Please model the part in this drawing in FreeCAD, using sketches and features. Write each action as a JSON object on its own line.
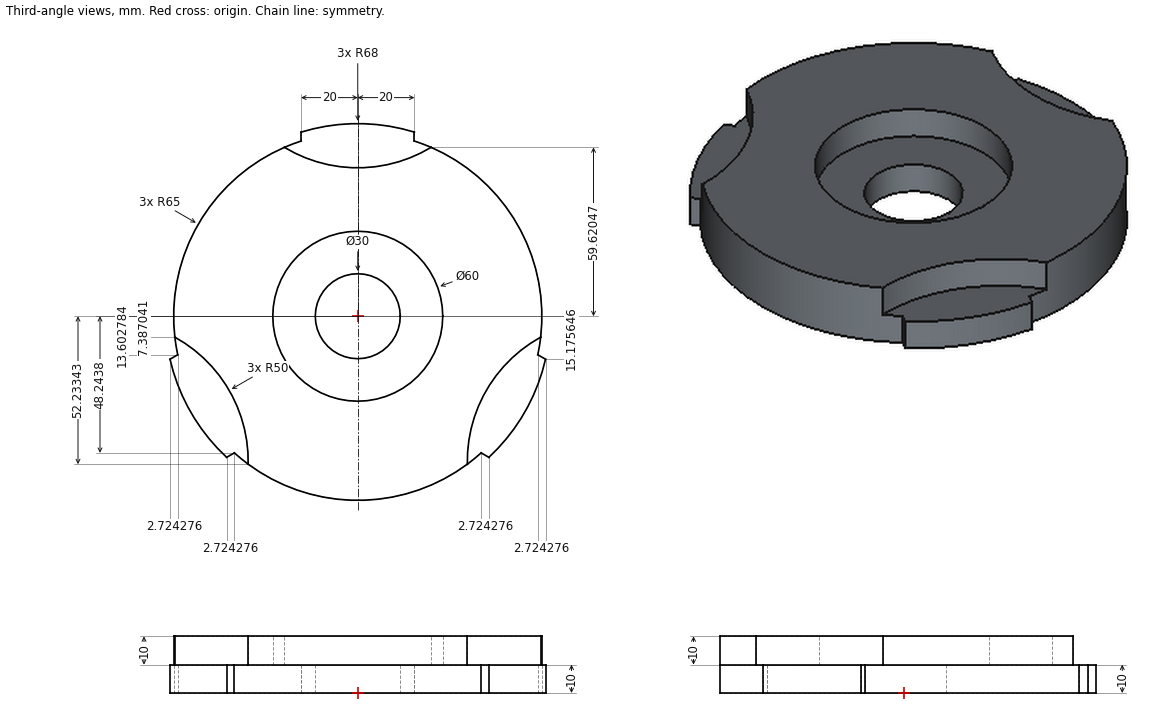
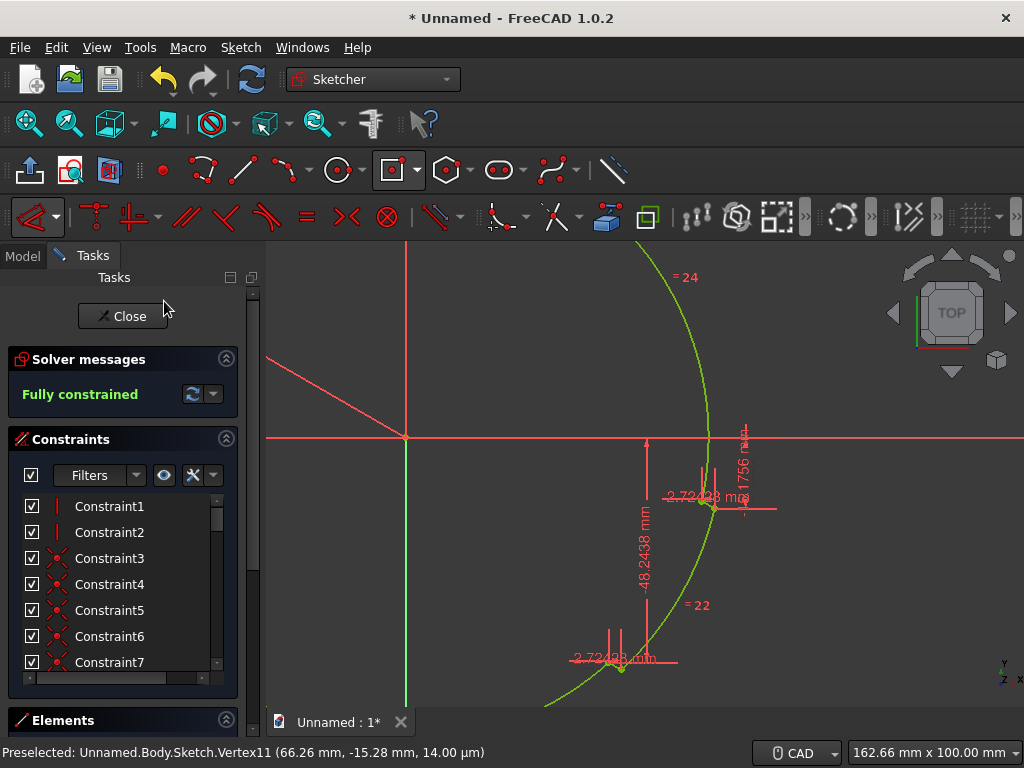
{"action": "left_click", "coordinate": [123, 316]}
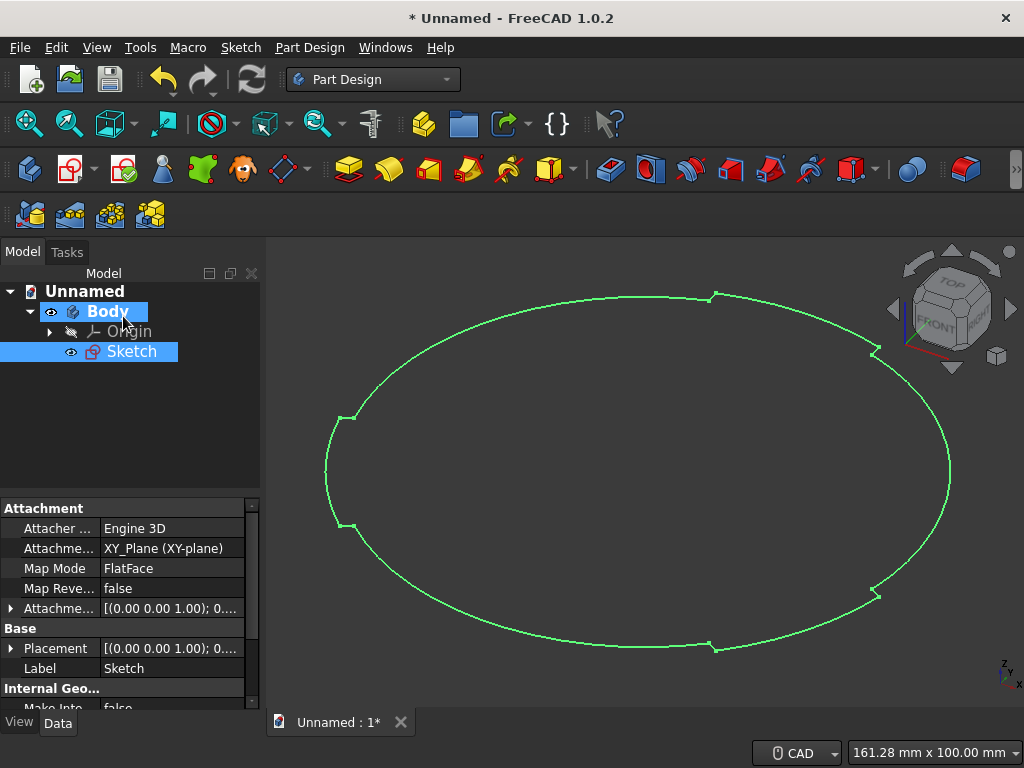
{"action": "left_click", "coordinate": [350, 170]}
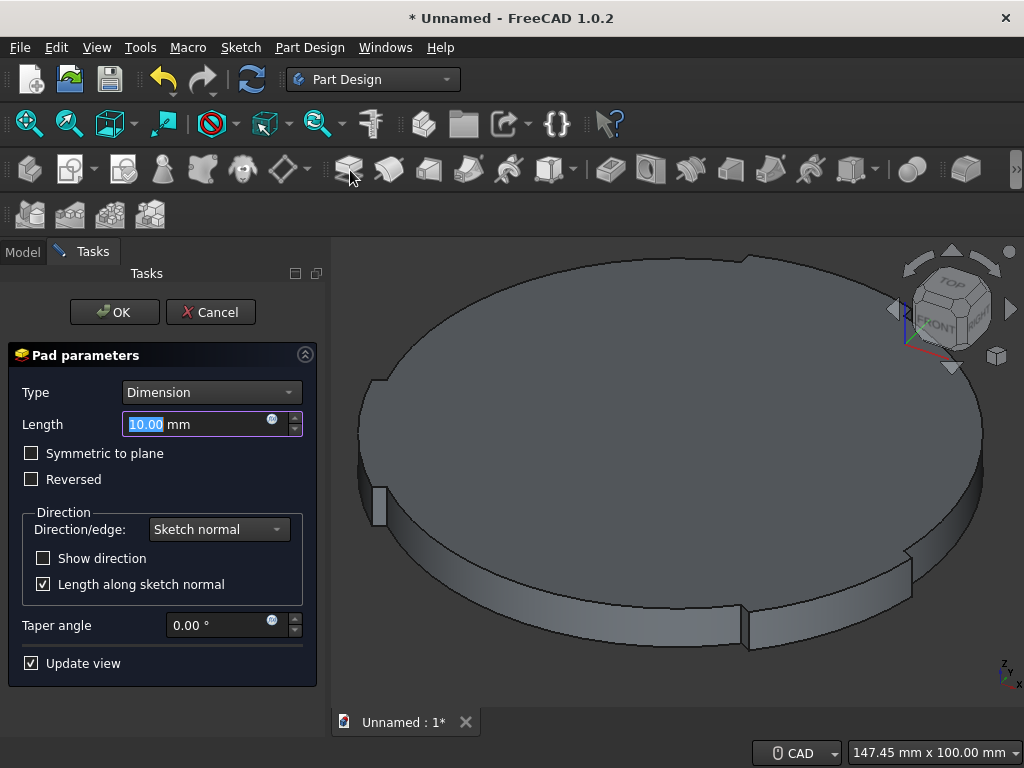
{"action": "type", "text": "10"}
{"action": "key", "text": "Tab"}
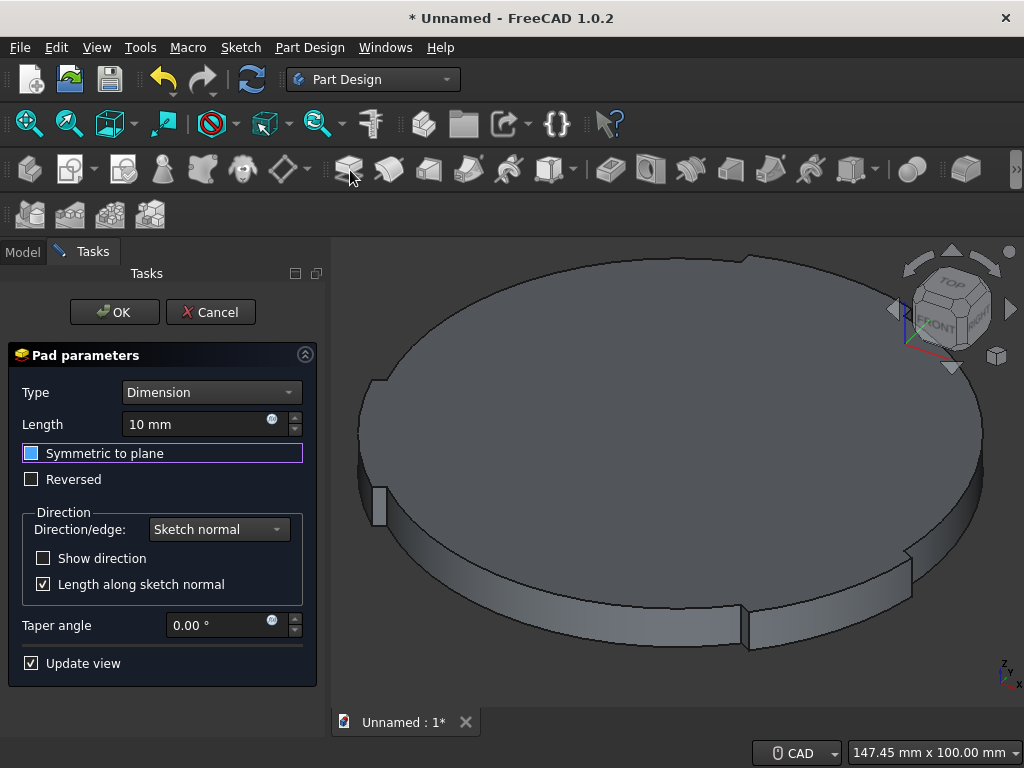
{"action": "left_click", "coordinate": [115, 312]}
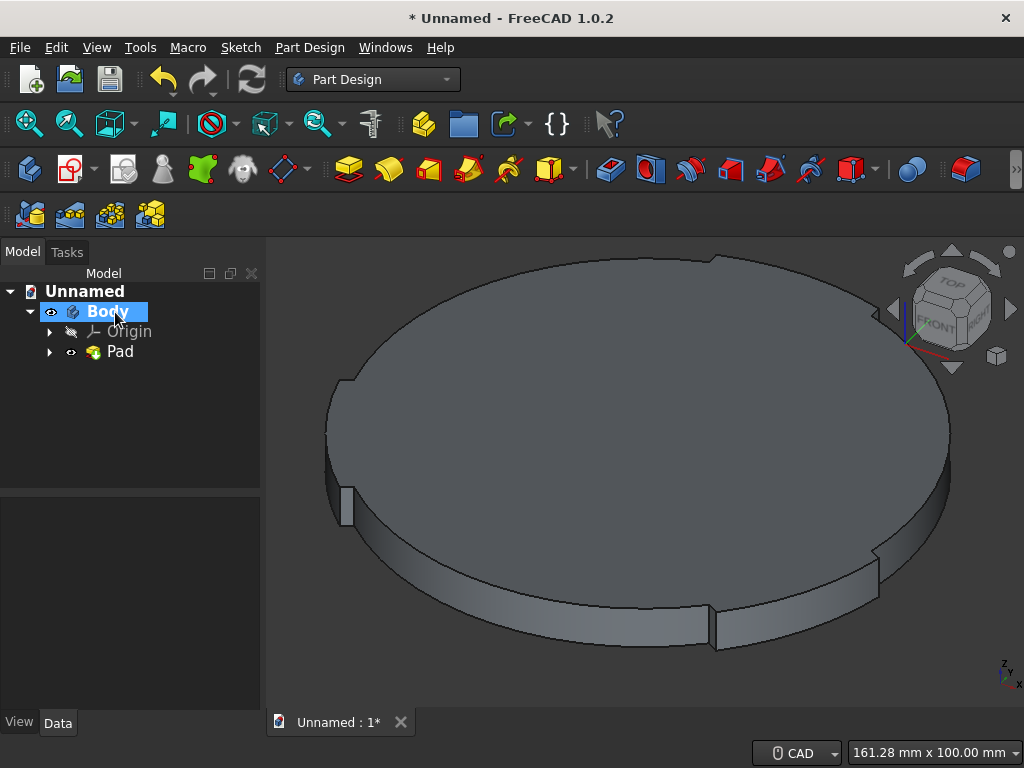
{"action": "left_click", "coordinate": [30, 124]}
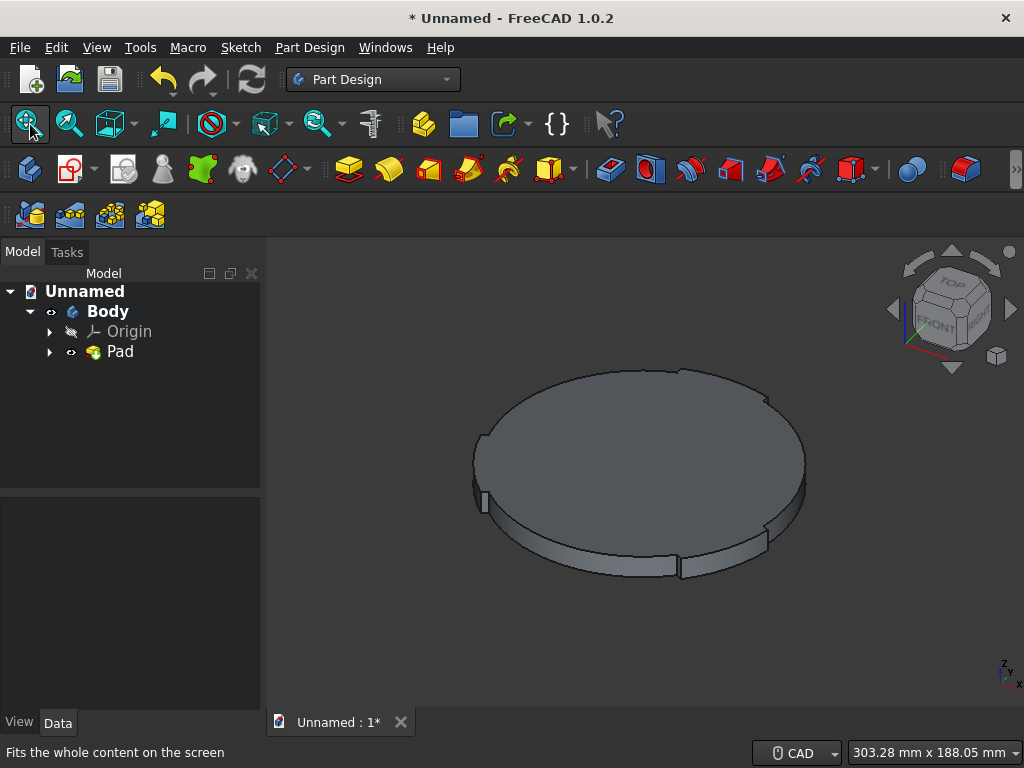
{"action": "left_click", "coordinate": [645, 461]}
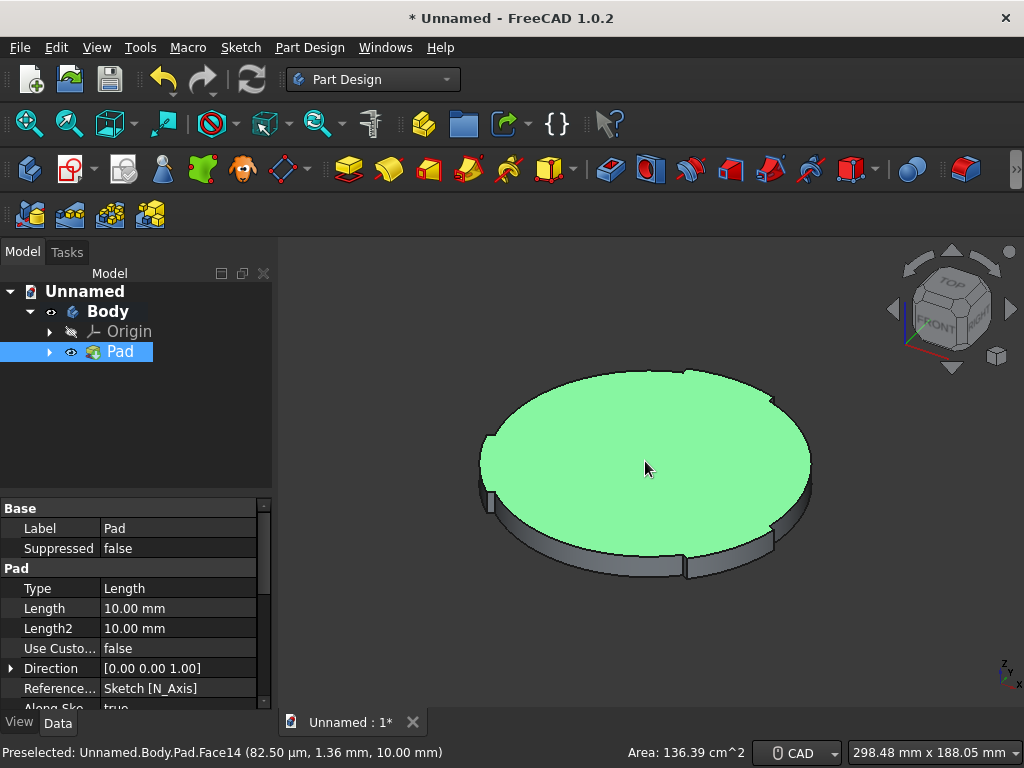
{"action": "left_click", "coordinate": [70, 170]}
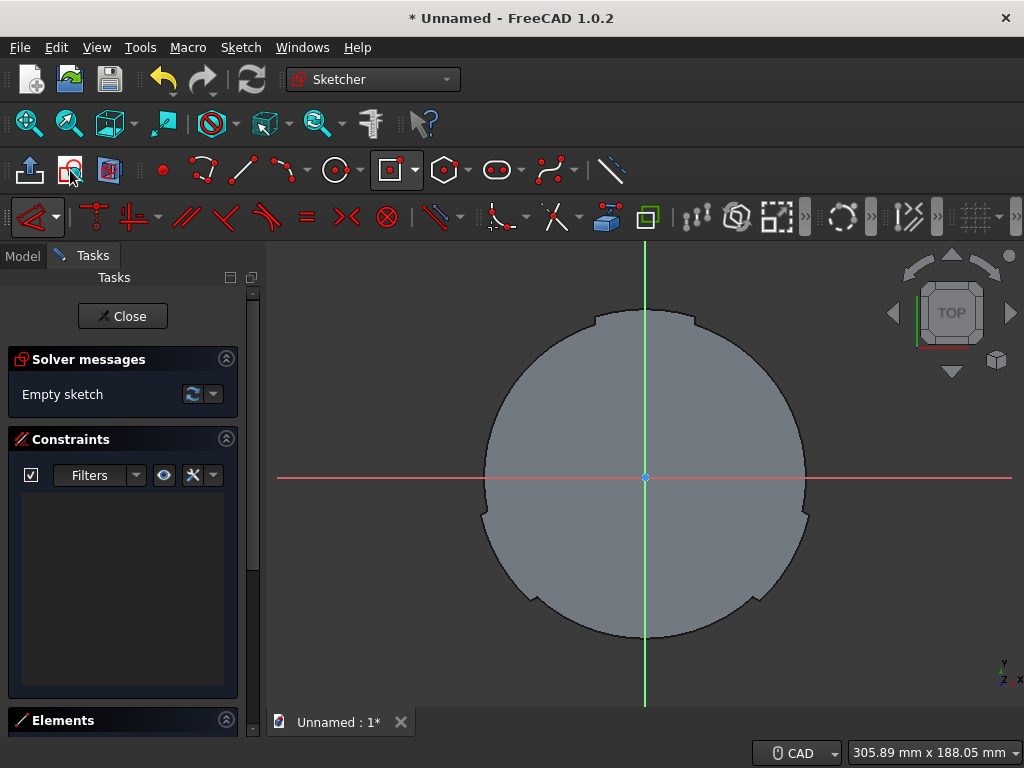
{"action": "left_click", "coordinate": [284, 170]}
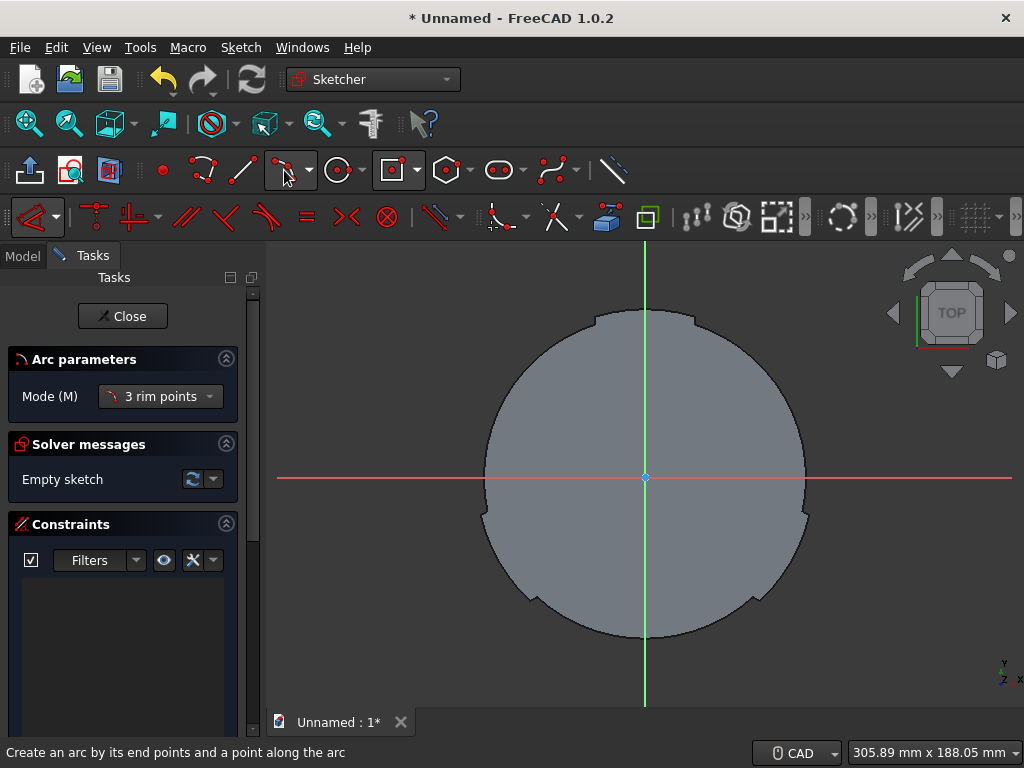
{"action": "left_click", "coordinate": [485, 496]}
{"action": "left_click", "coordinate": [549, 607]}
{"action": "left_click", "coordinate": [533, 543]}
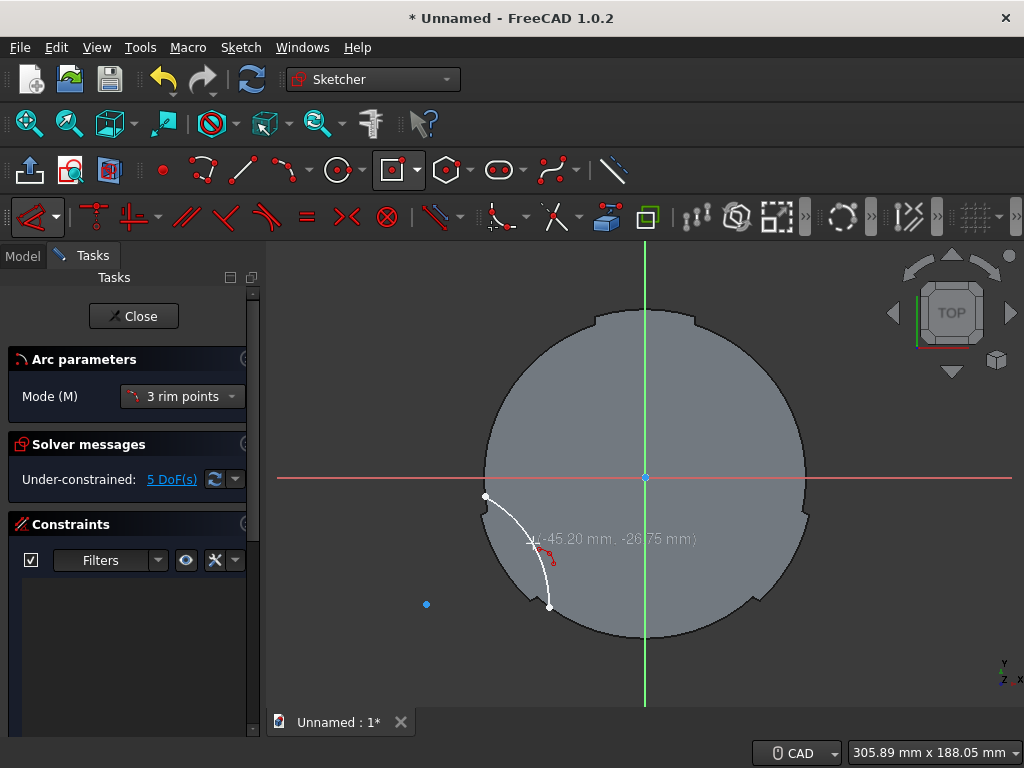
{"action": "left_click", "coordinate": [549, 608]}
{"action": "left_click", "coordinate": [741, 607]}
{"action": "left_click", "coordinate": [625, 637]}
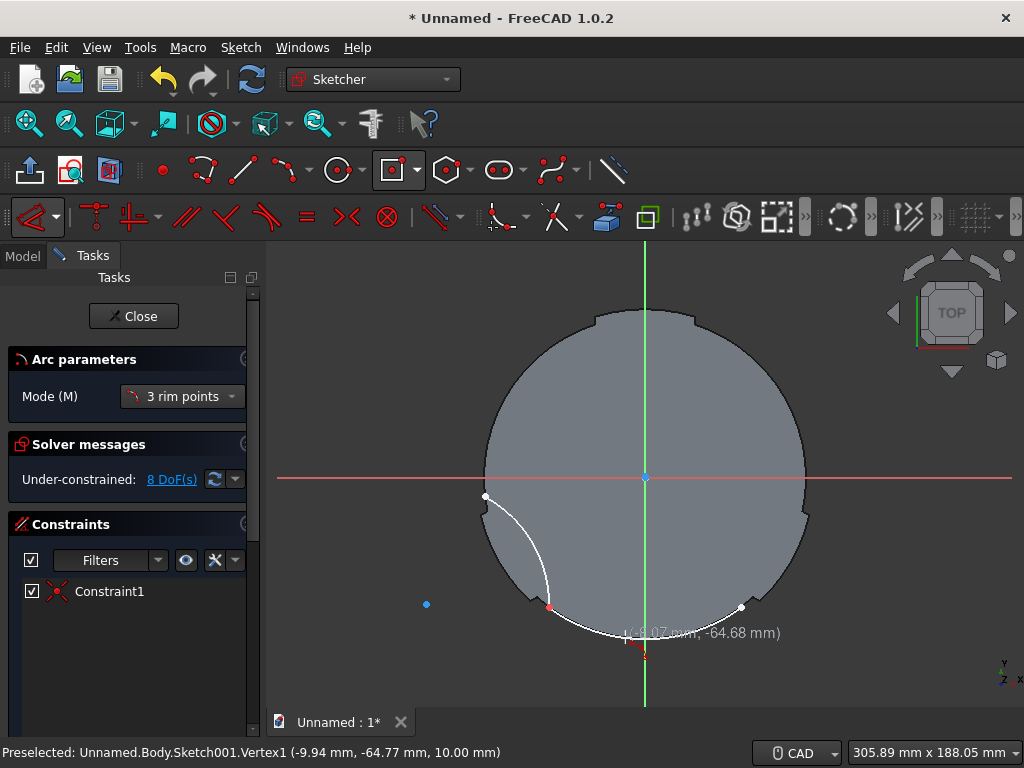
{"action": "left_click", "coordinate": [741, 608]}
{"action": "left_click", "coordinate": [805, 496]}
{"action": "left_click", "coordinate": [757, 543]}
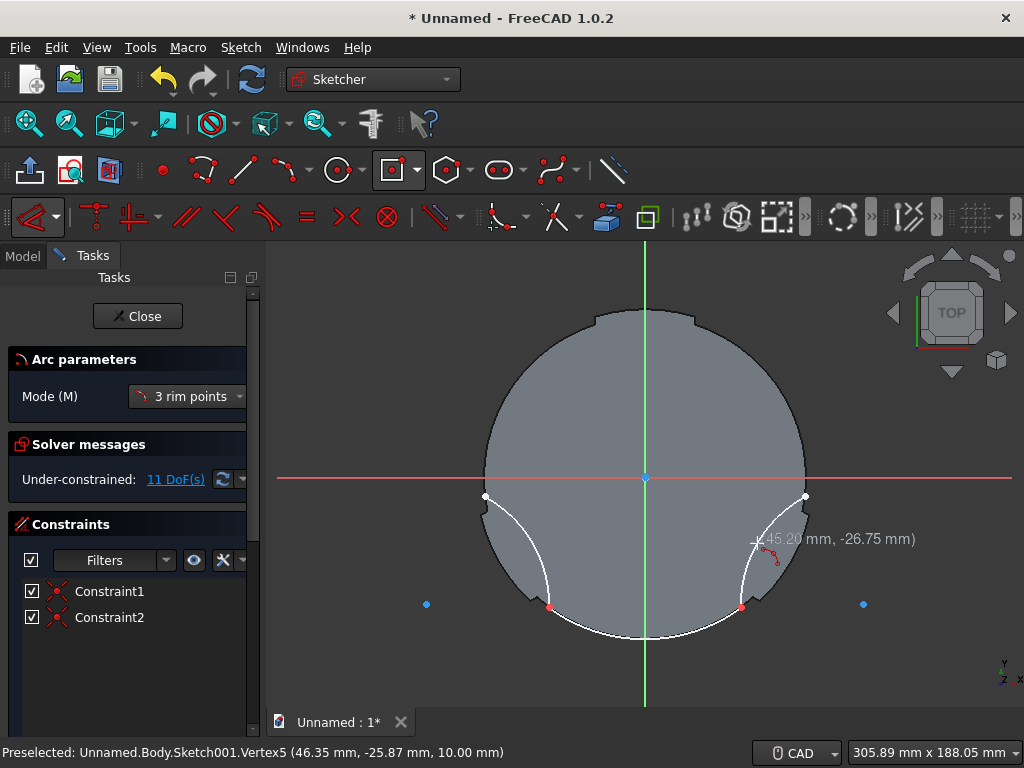
{"action": "left_click", "coordinate": [805, 497]}
{"action": "left_click", "coordinate": [709, 330]}
{"action": "left_click", "coordinate": [784, 397]}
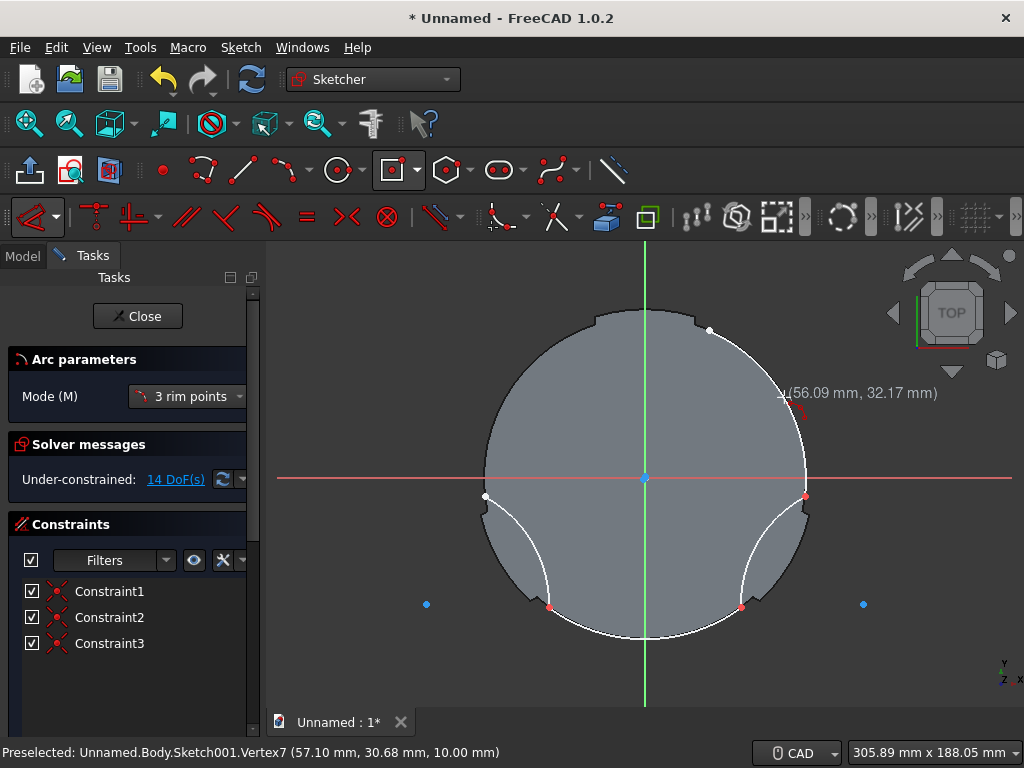
{"action": "left_click", "coordinate": [709, 331]}
{"action": "left_click", "coordinate": [581, 330]}
{"action": "left_click", "coordinate": [618, 345]}